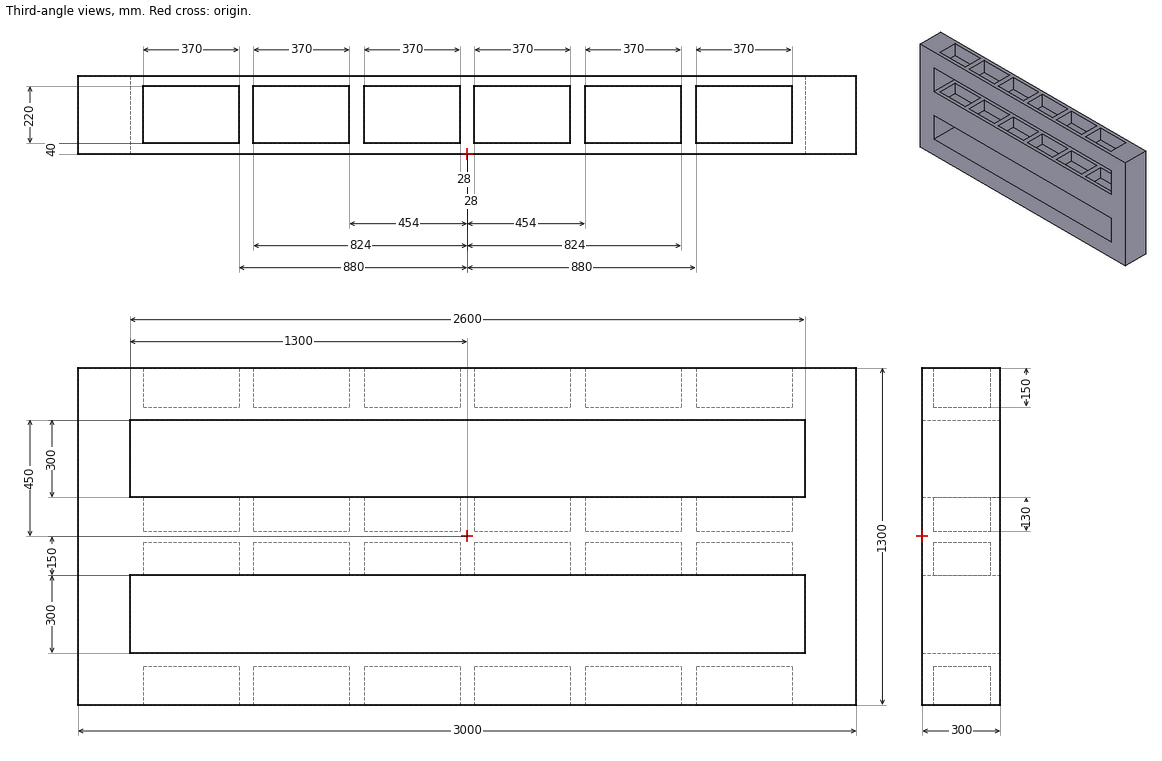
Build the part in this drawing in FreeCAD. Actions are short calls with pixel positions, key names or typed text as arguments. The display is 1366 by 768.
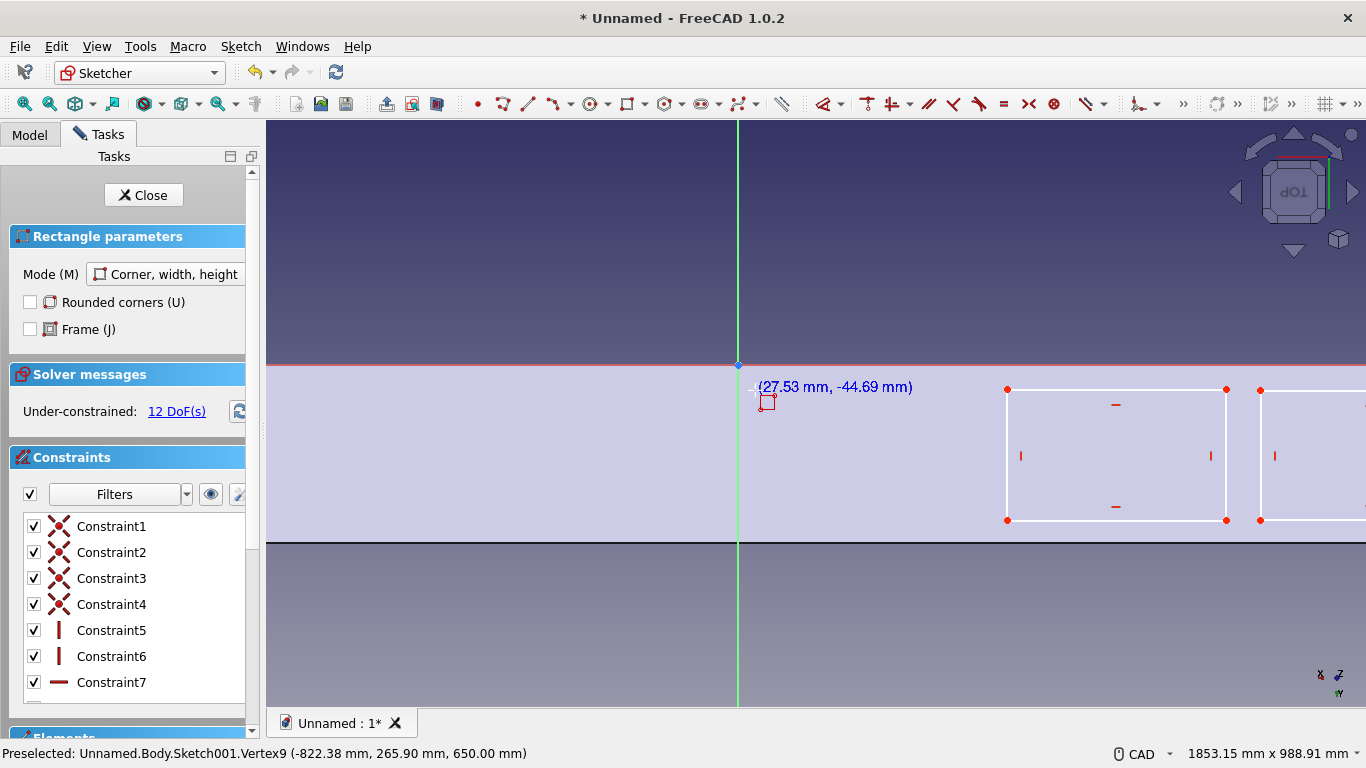
click(755, 389)
click(974, 519)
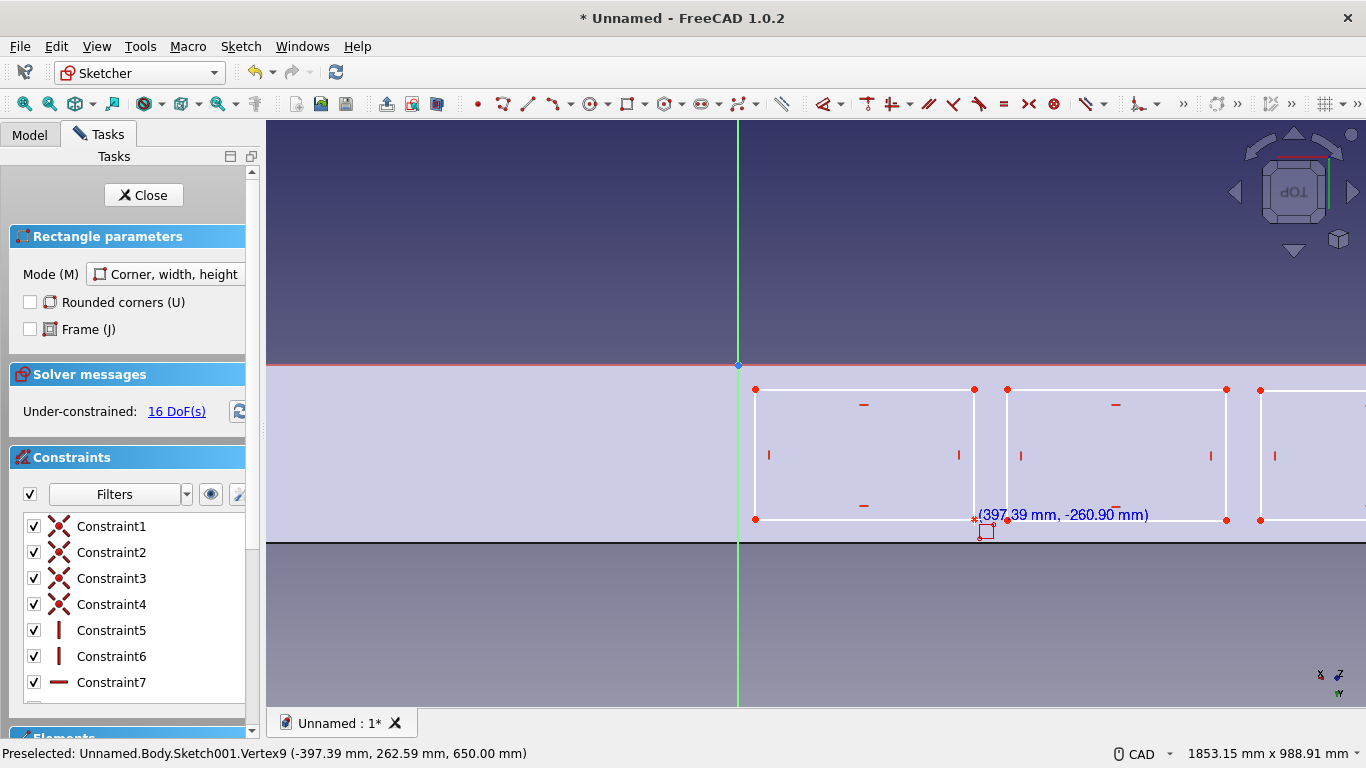
click(502, 389)
click(721, 519)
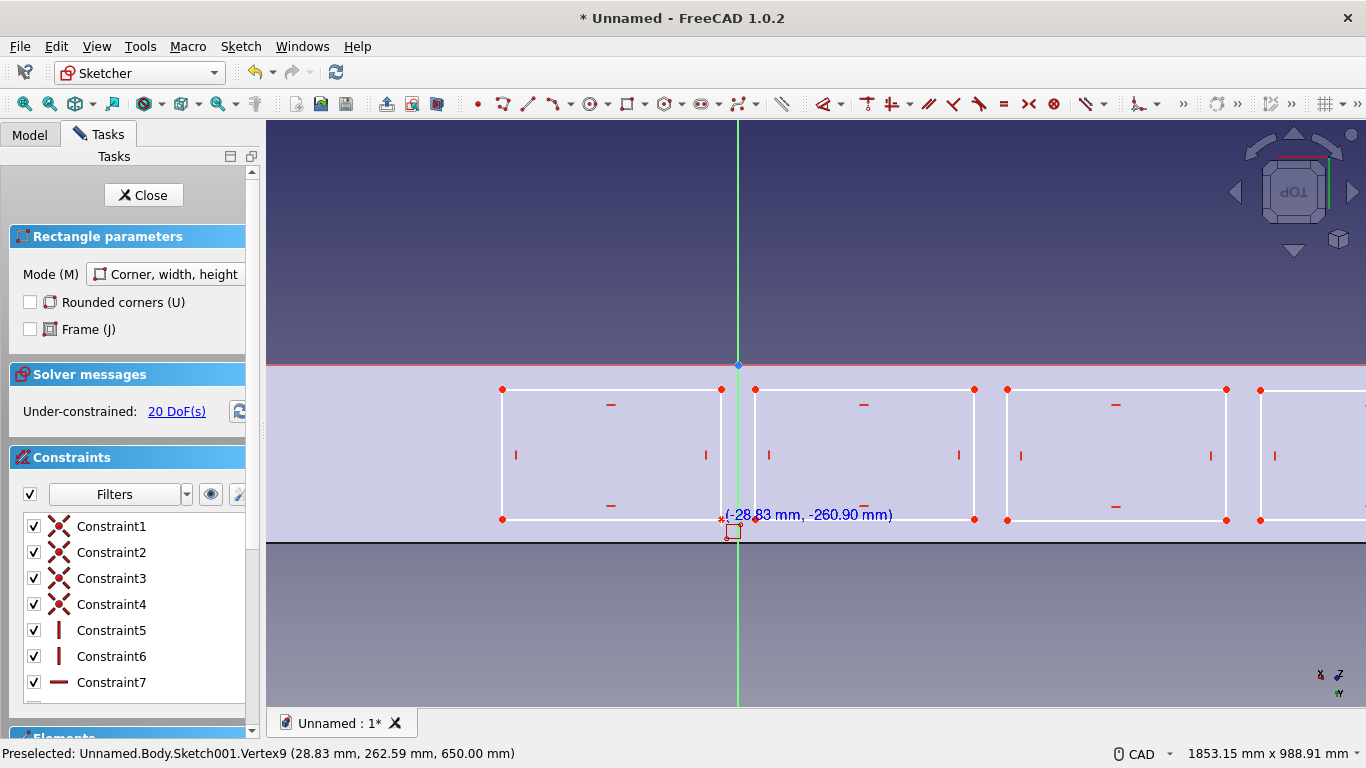
scroll(755, 390, down, 4)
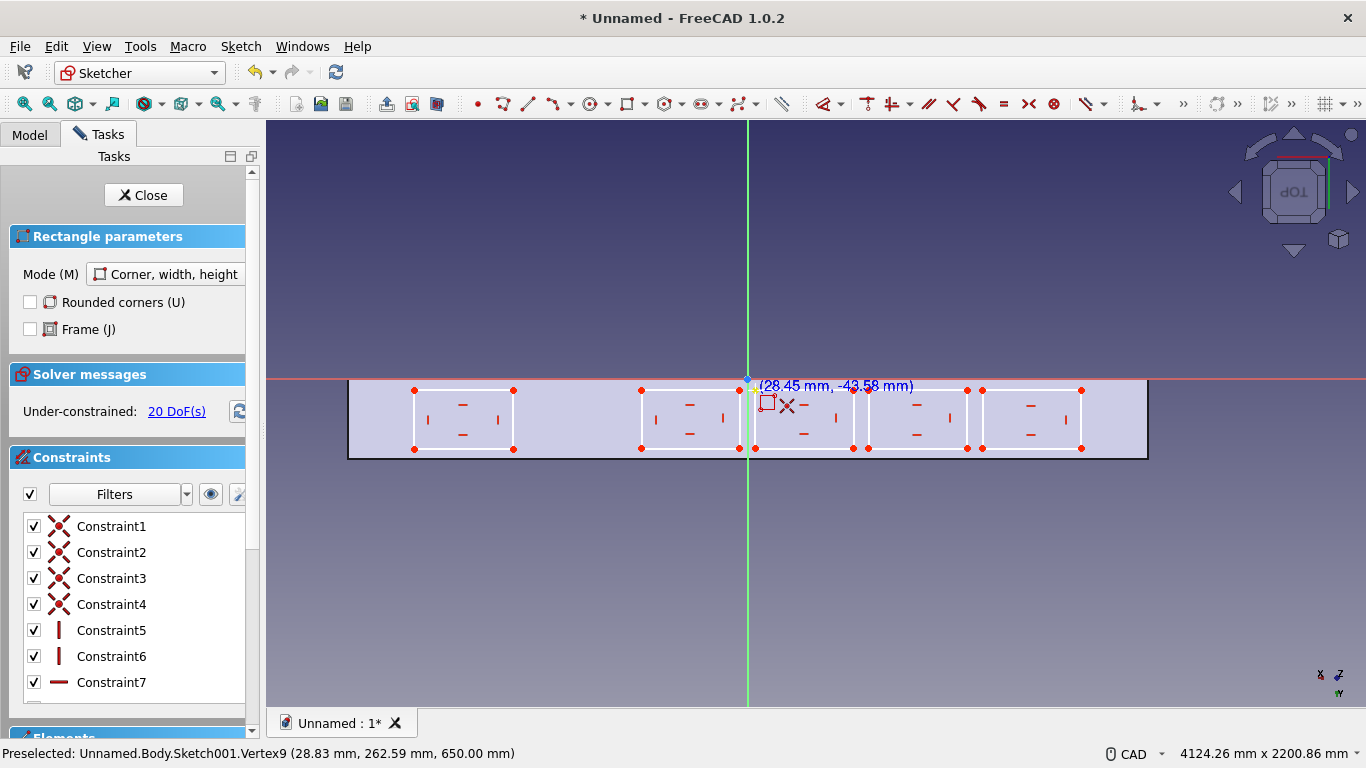
scroll(528, 390, up, 2)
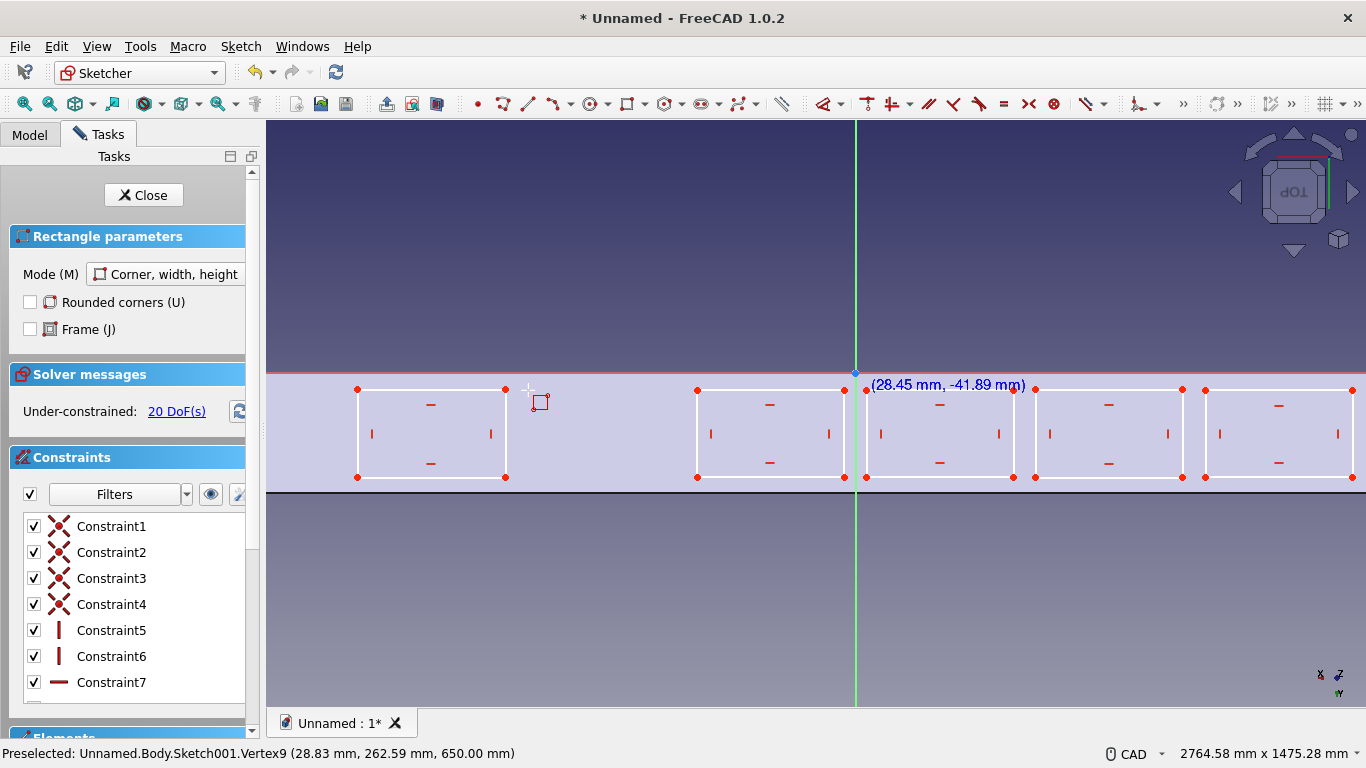
click(528, 389)
click(675, 477)
key(Escape)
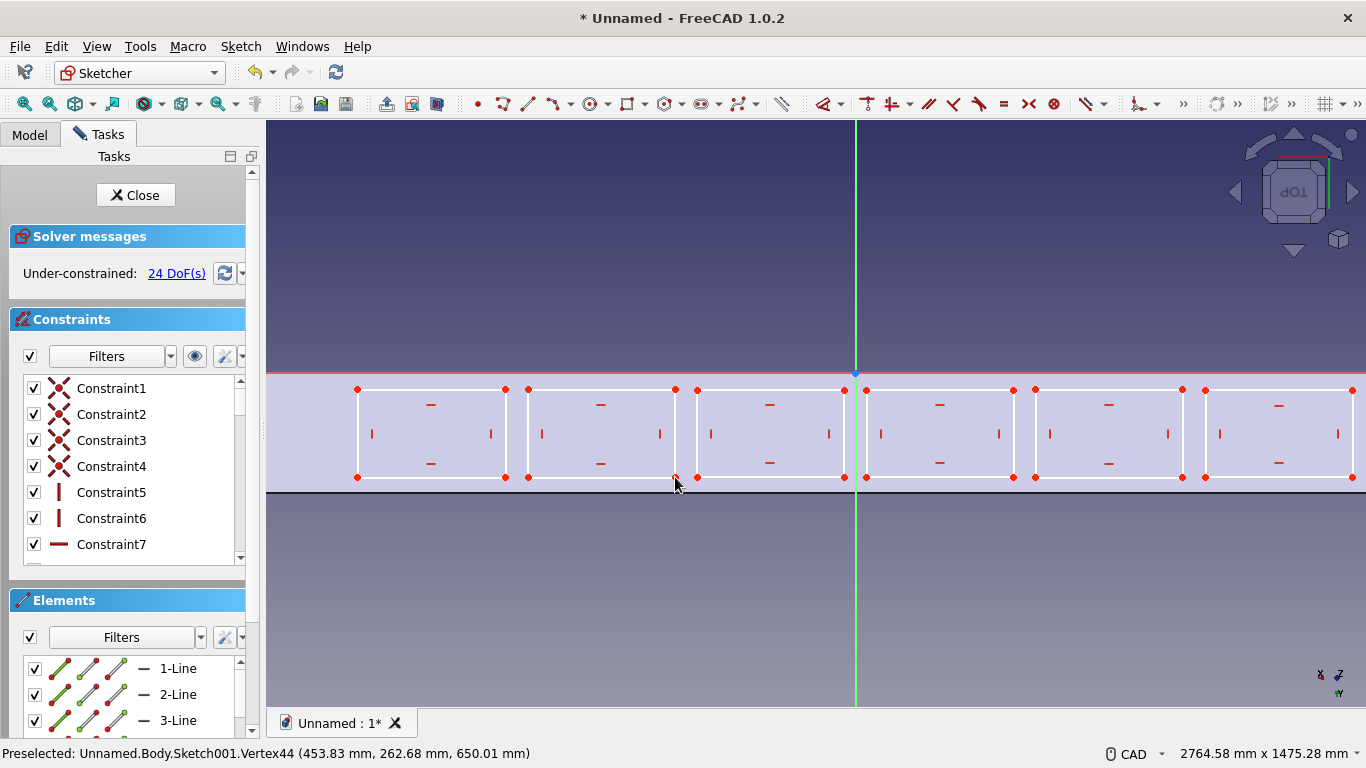
key(d)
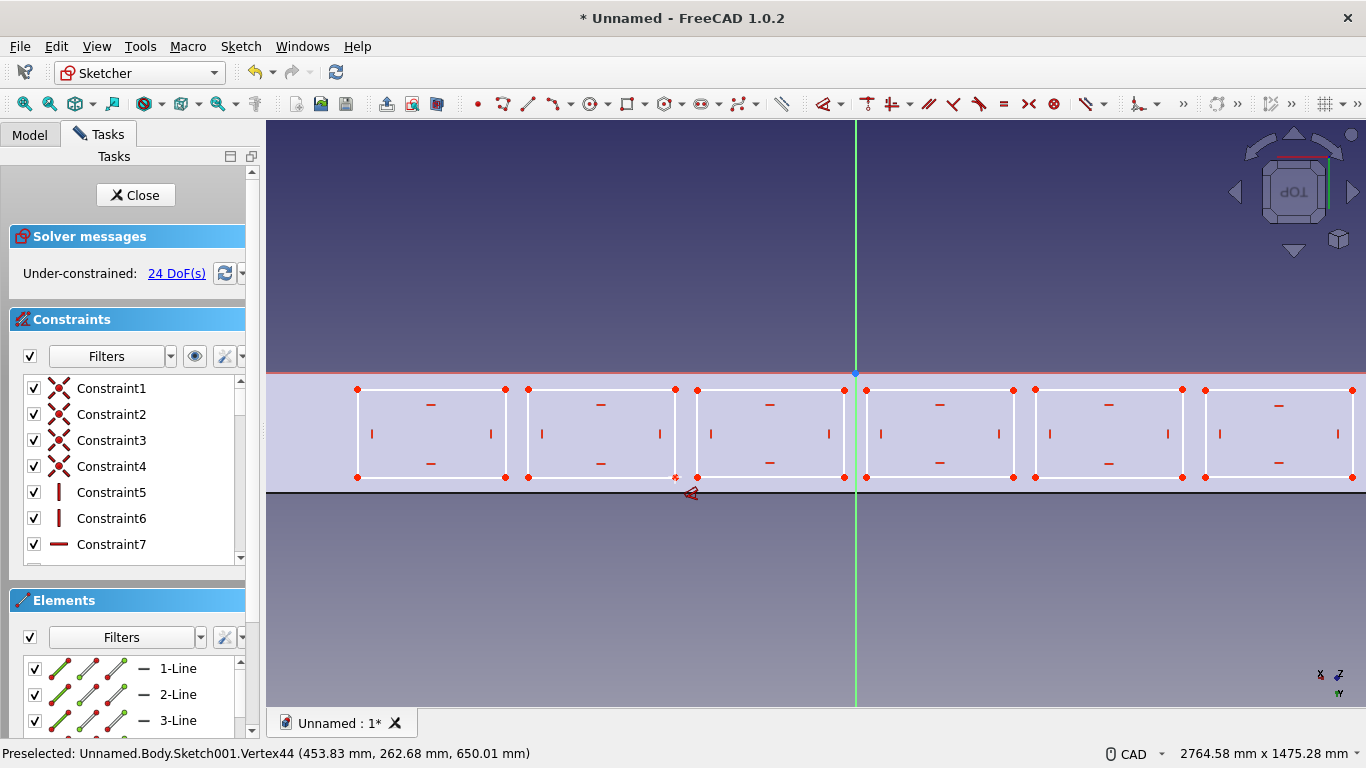
scroll(528, 390, down, 2)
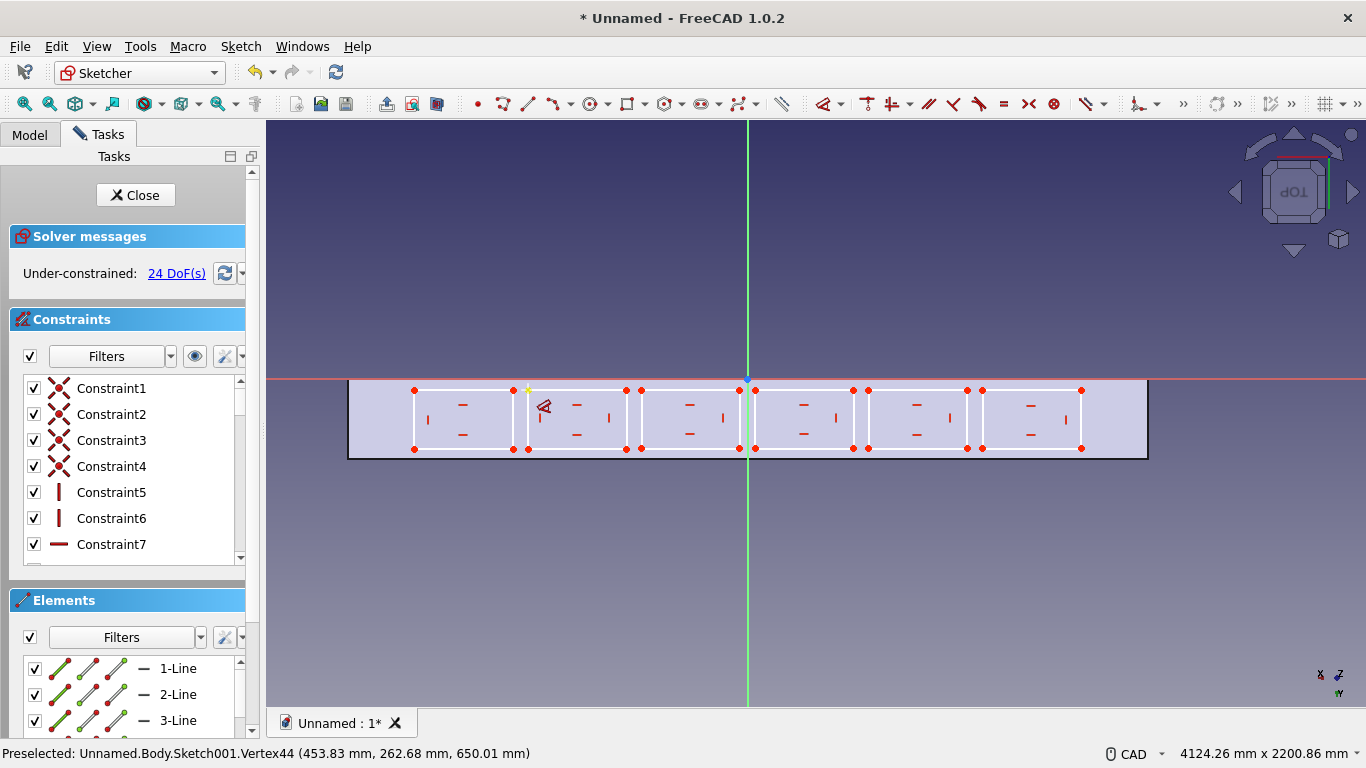
click(983, 408)
click(1017, 420)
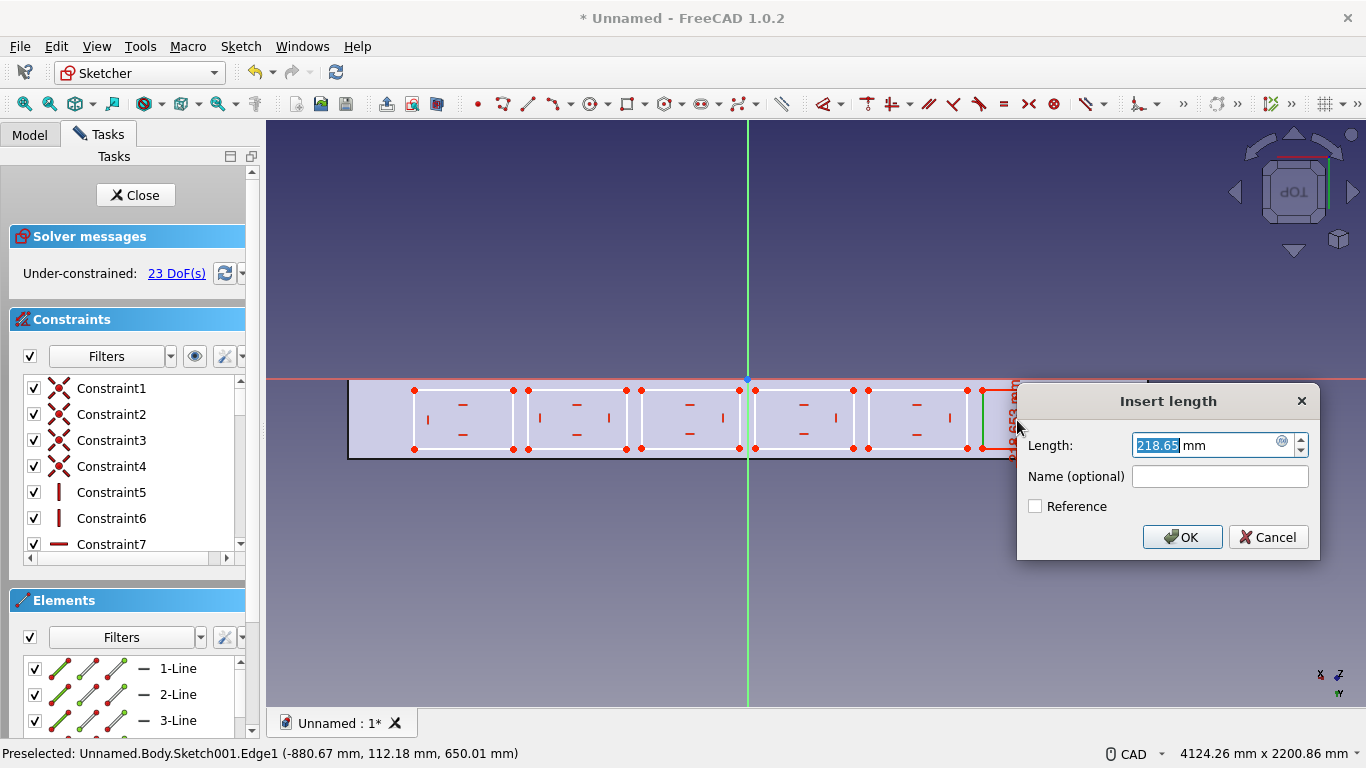
text(220)
key(Return)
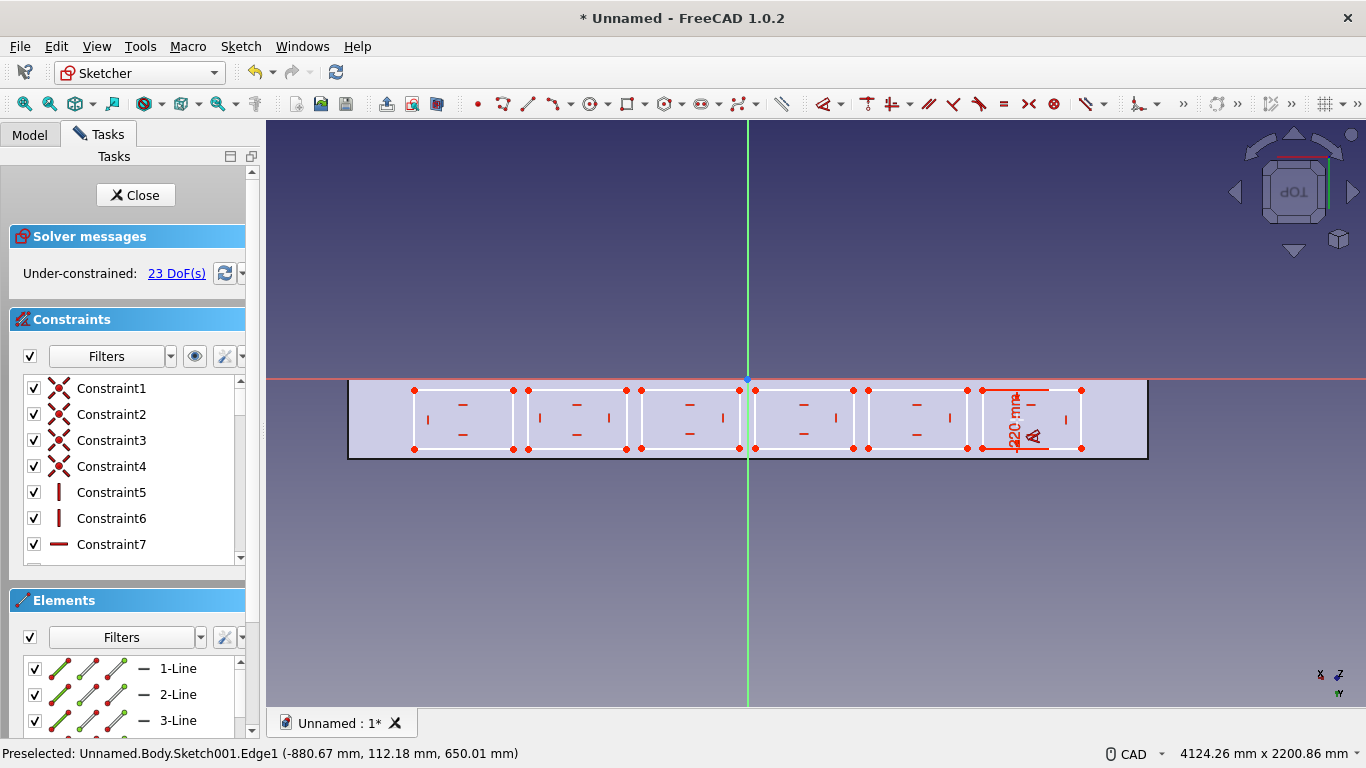
click(1012, 449)
click(1032, 483)